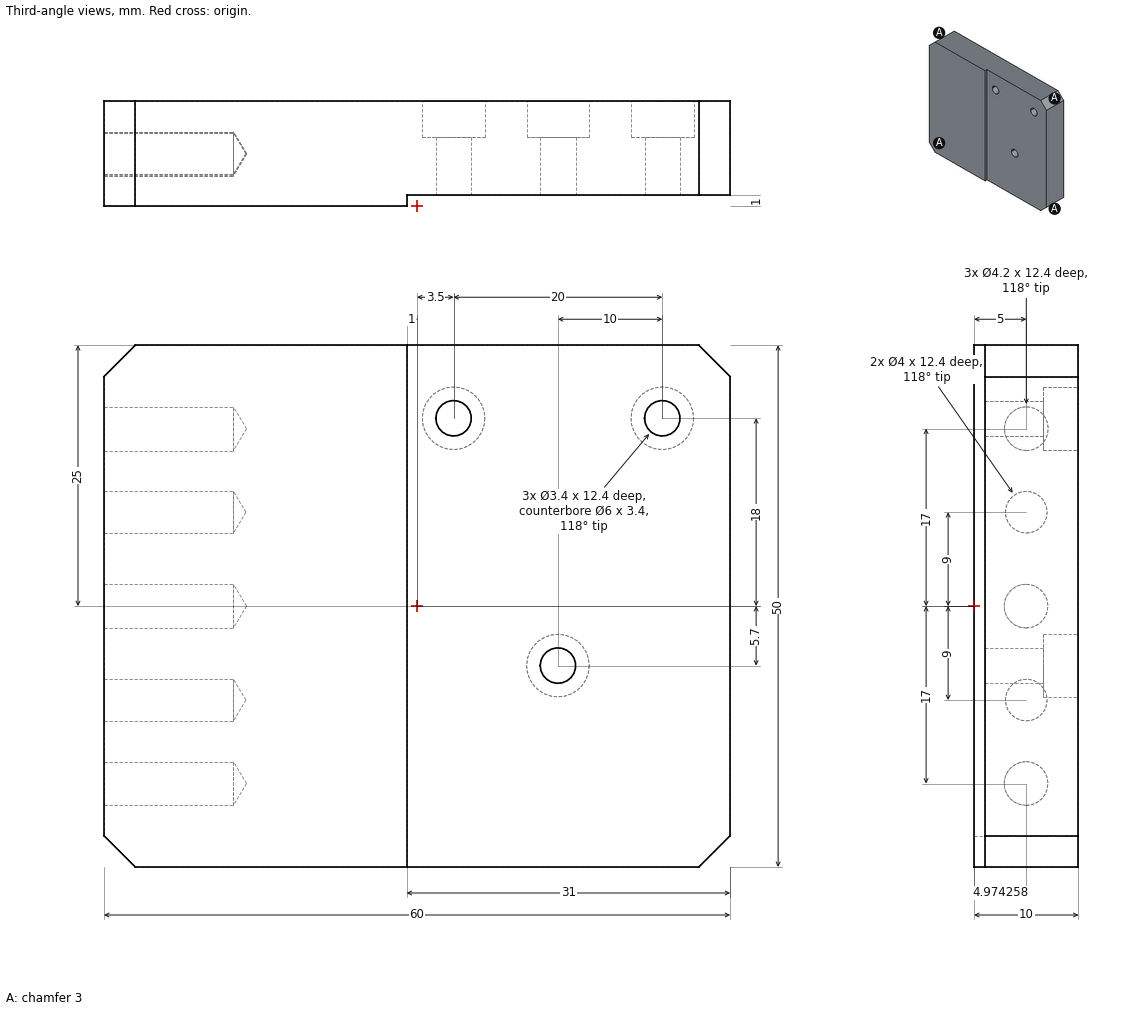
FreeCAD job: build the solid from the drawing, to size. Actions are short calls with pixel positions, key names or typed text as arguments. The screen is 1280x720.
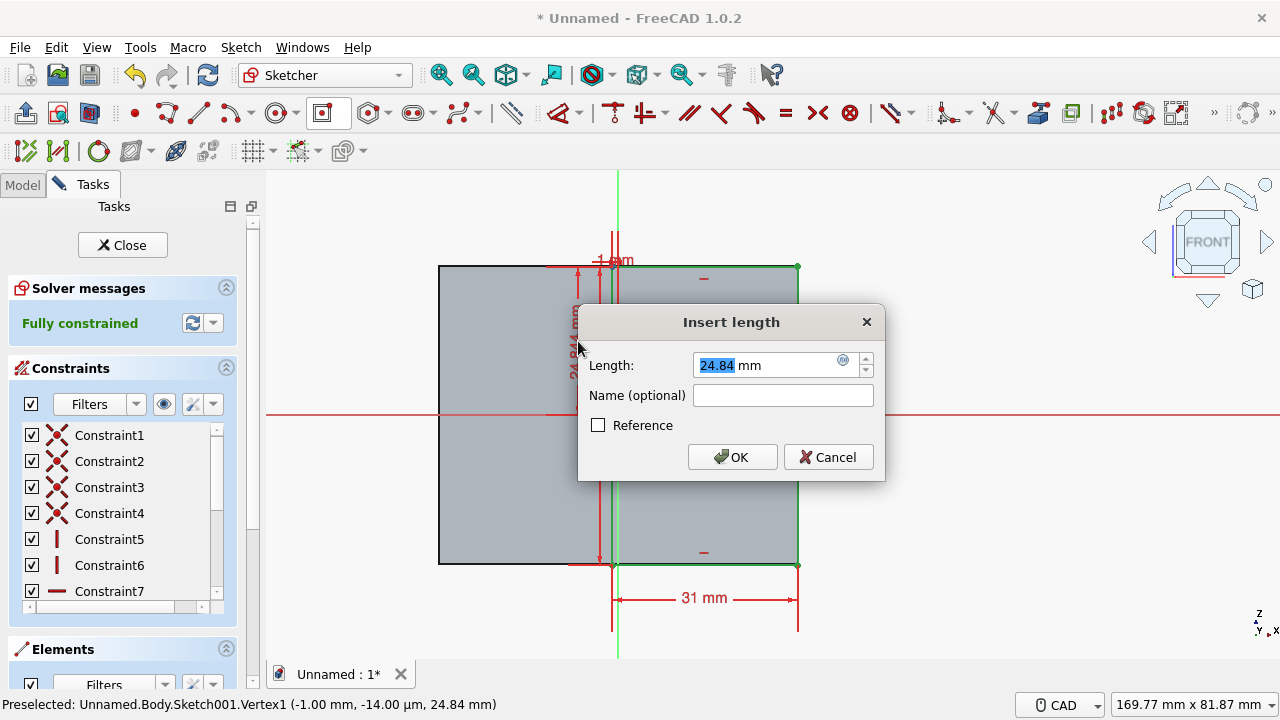
text(25)
key(Return)
key(Escape)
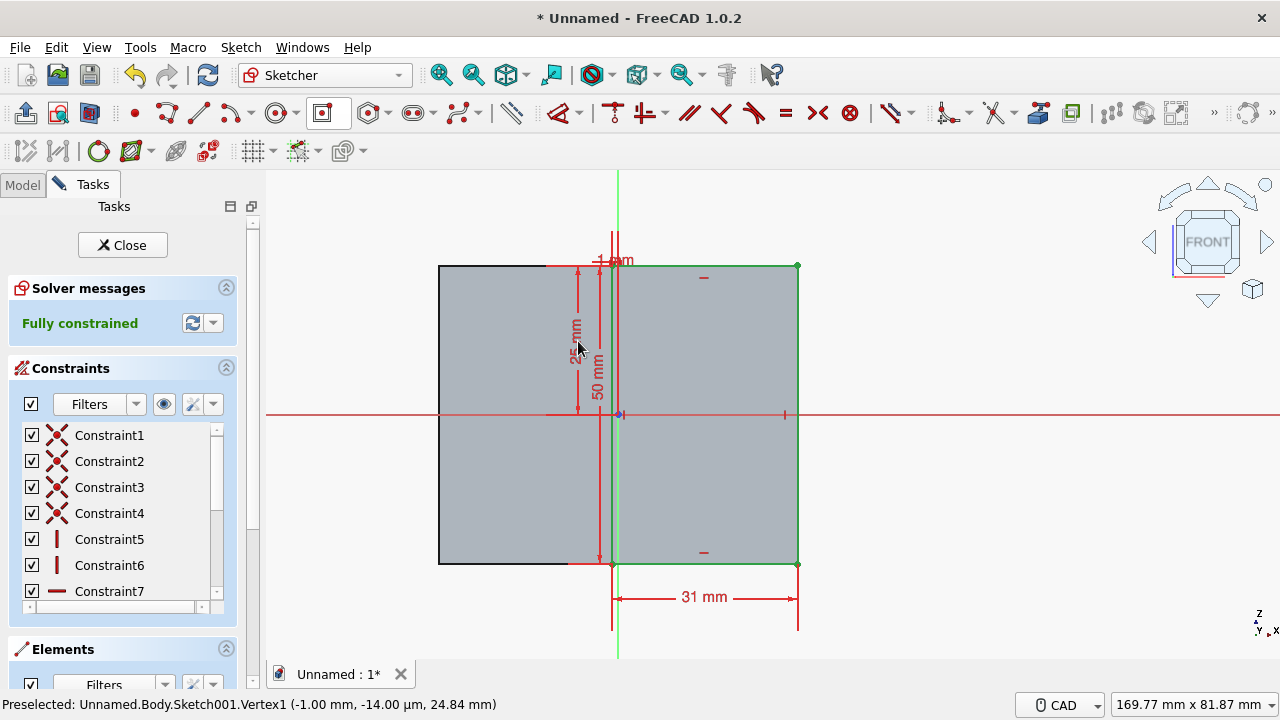
click(123, 245)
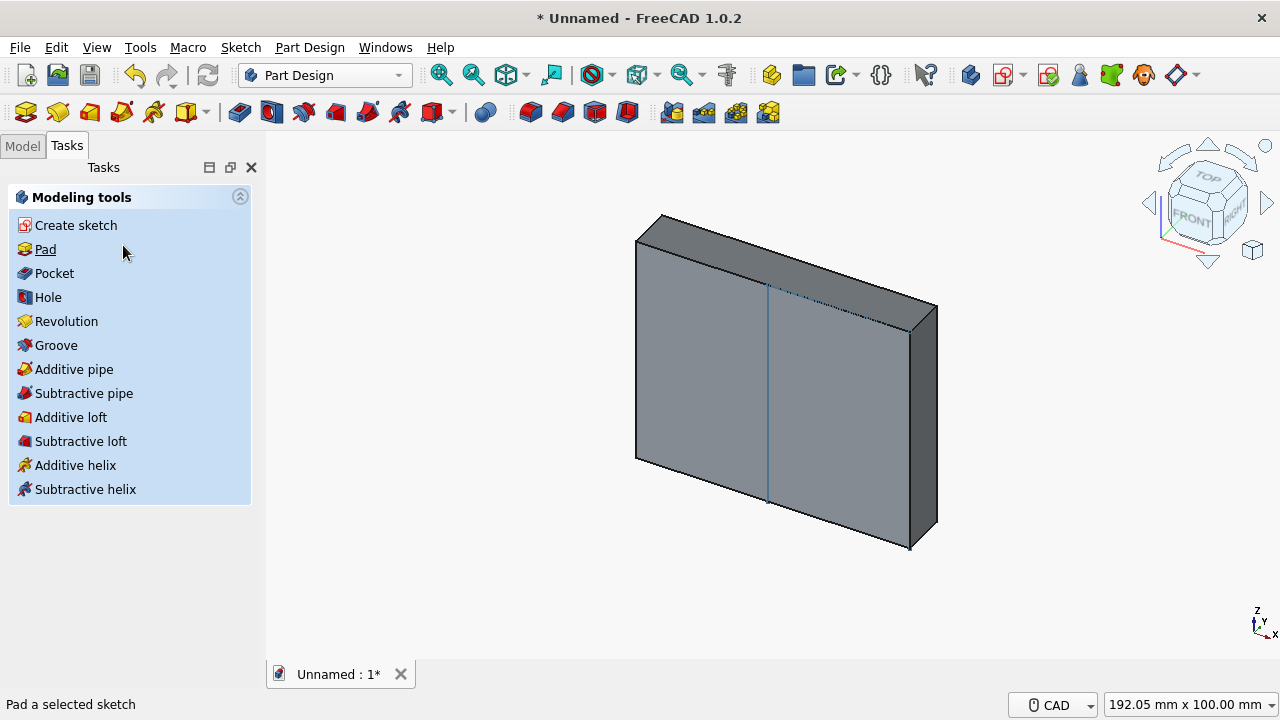
click(240, 112)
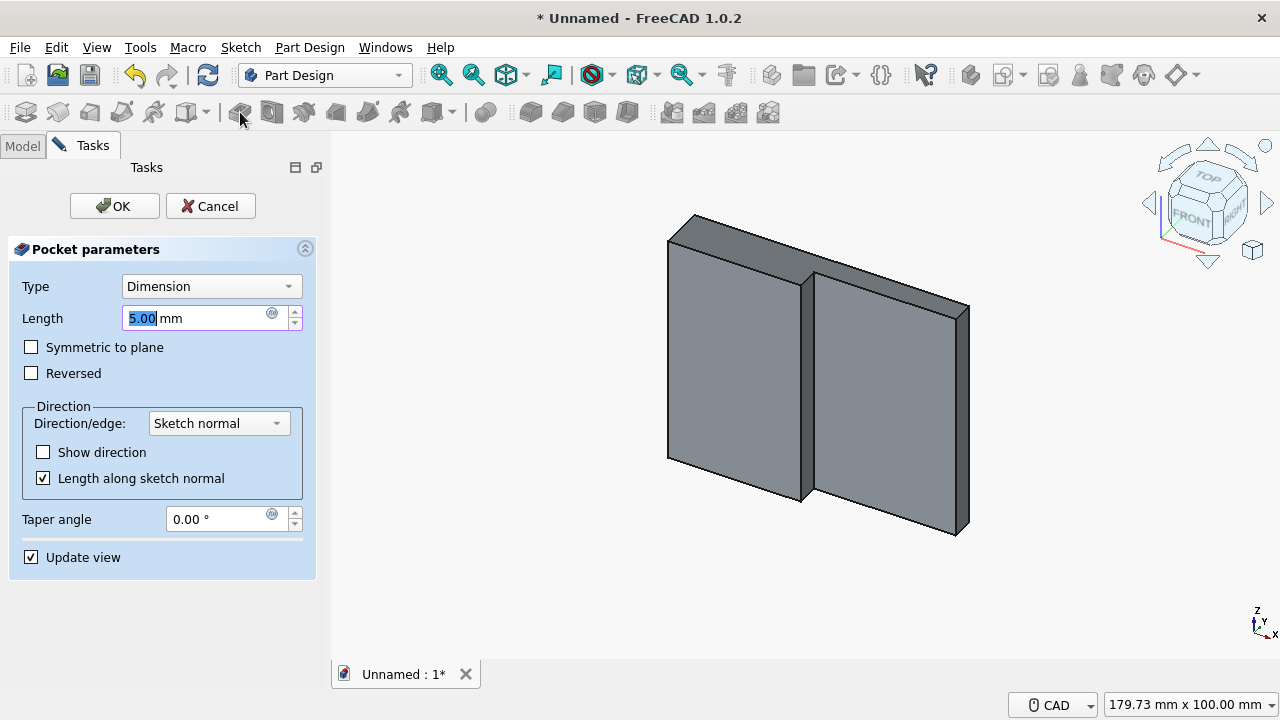
text(1)
key(Tab)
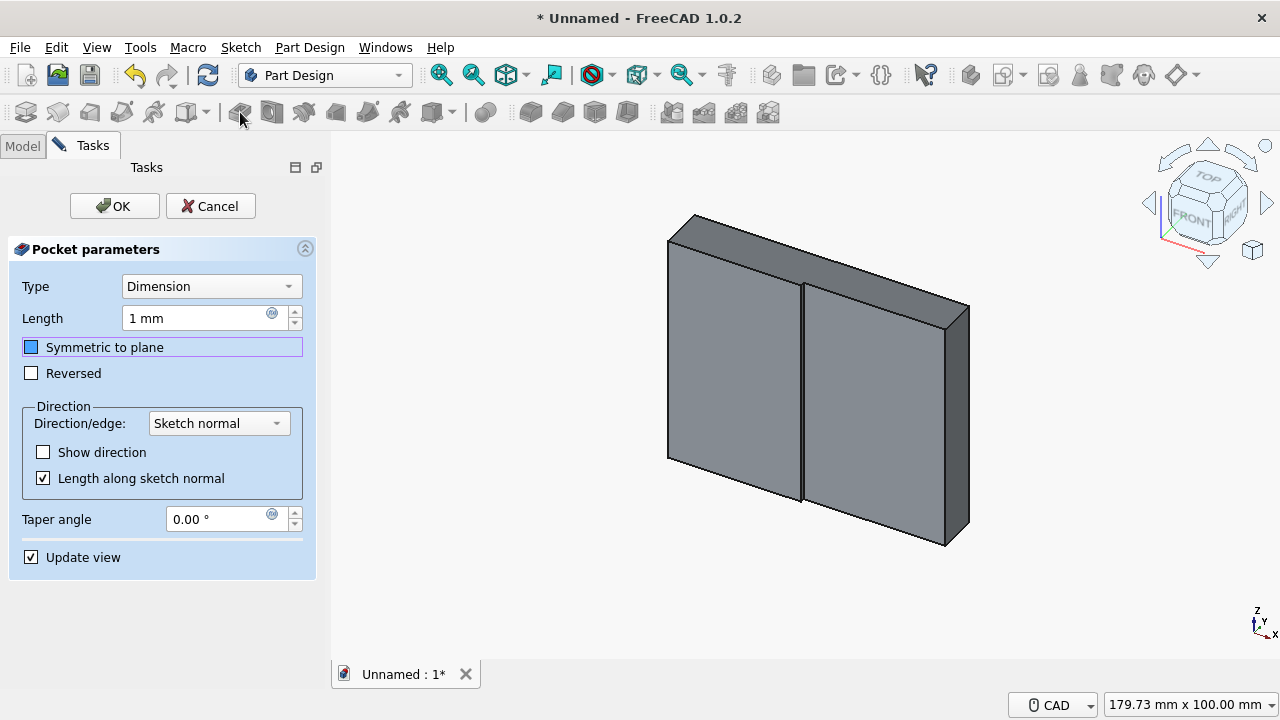
click(115, 206)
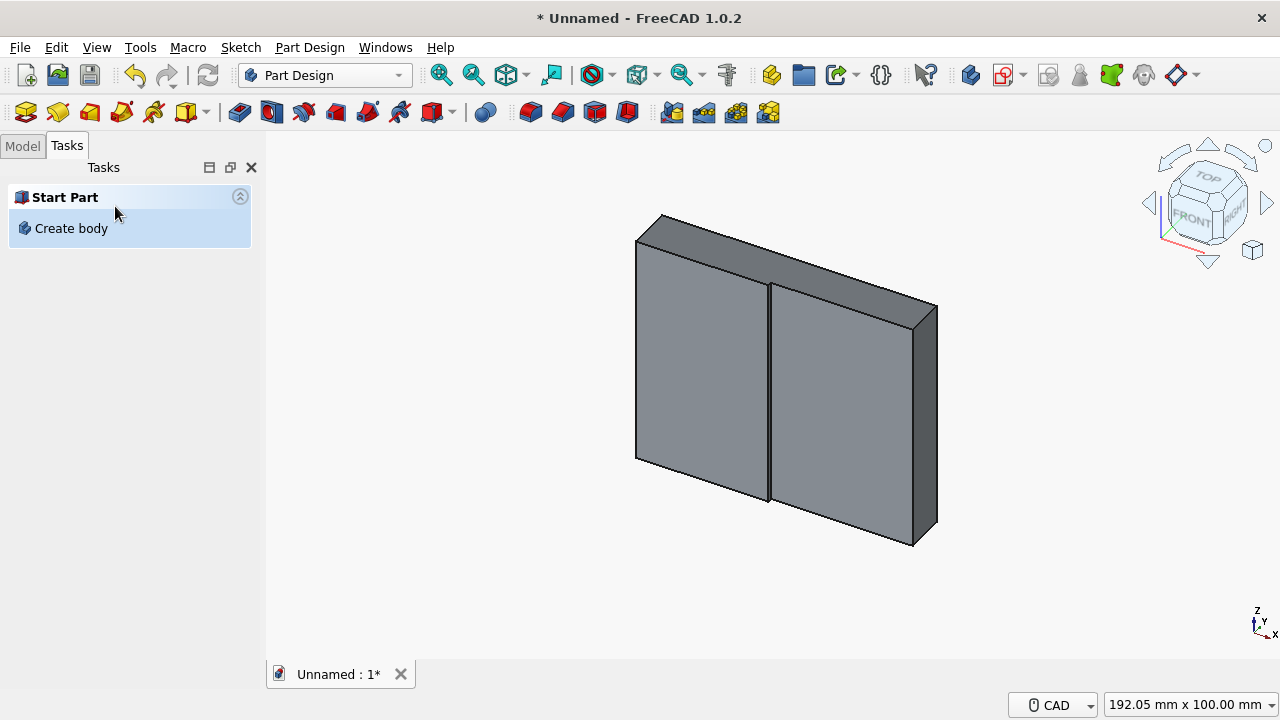
click(925, 317)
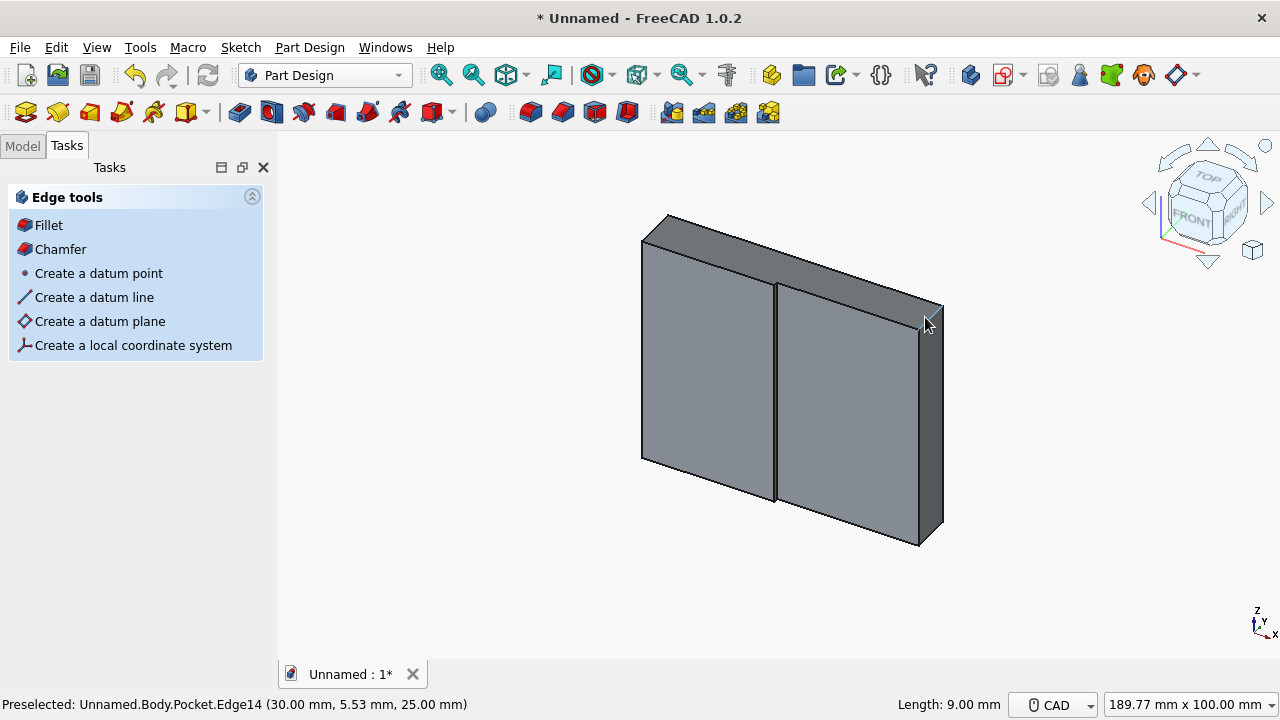
key(0)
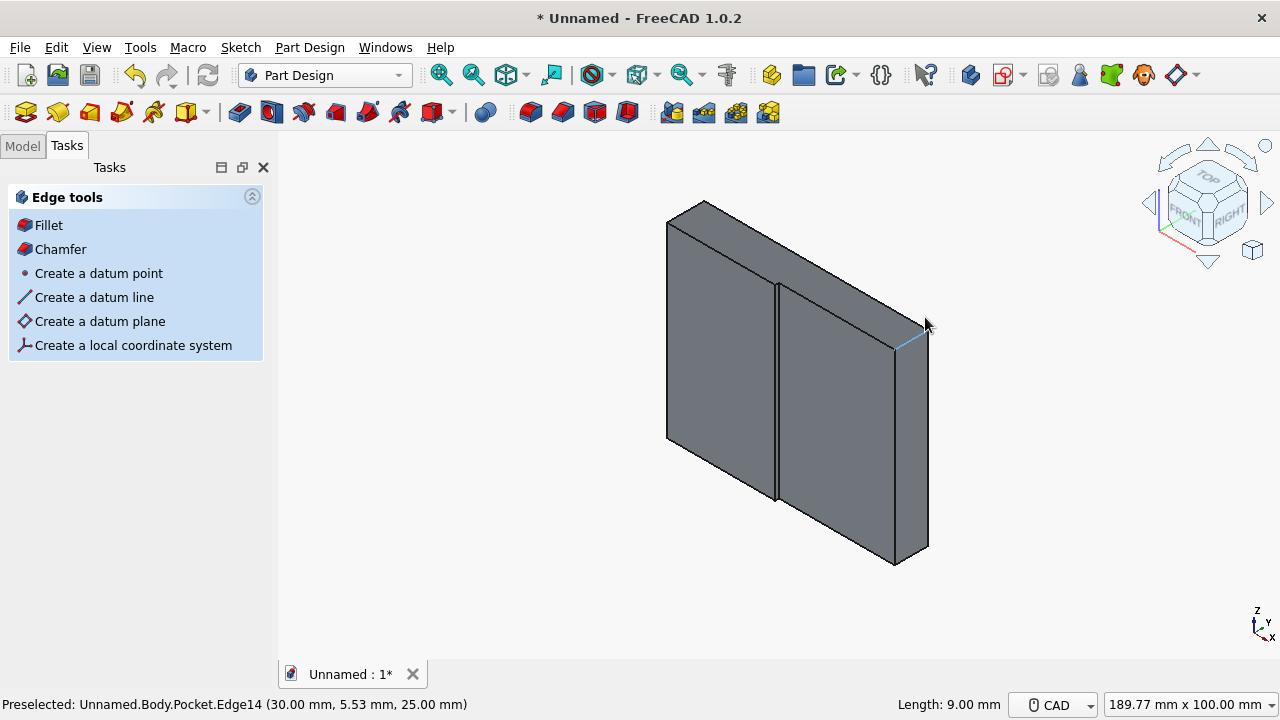
key(2)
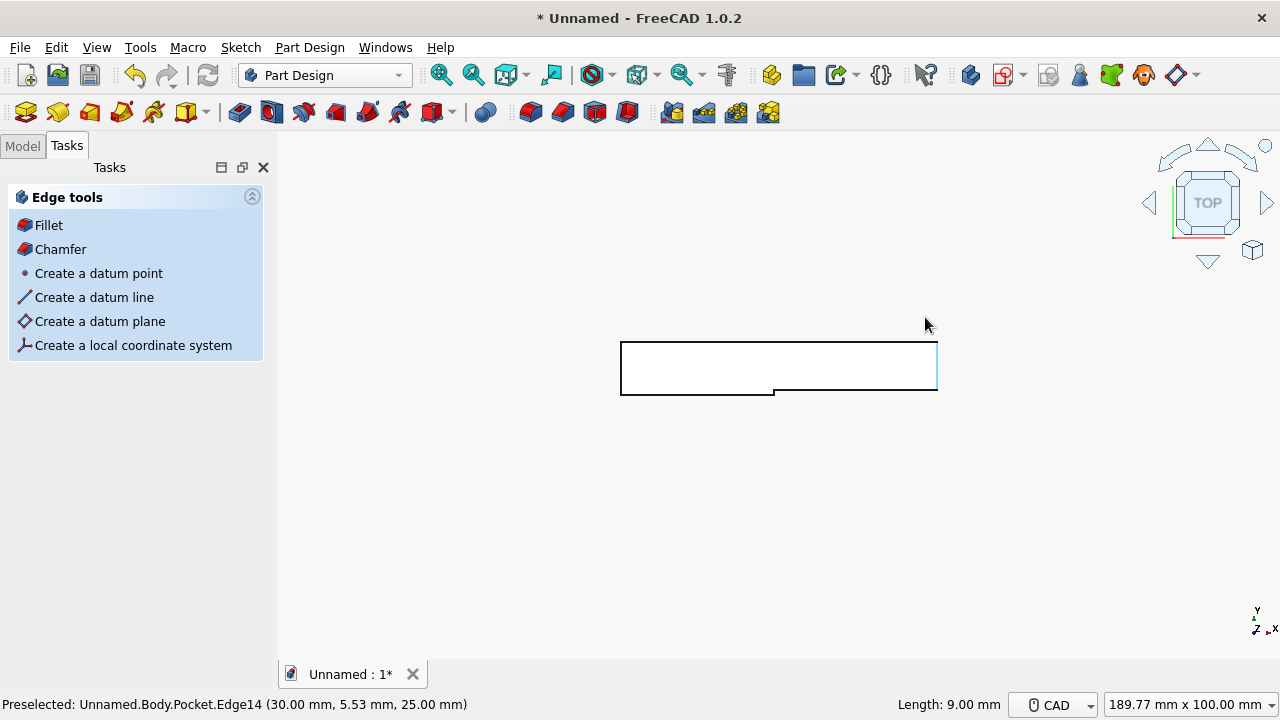
click(442, 76)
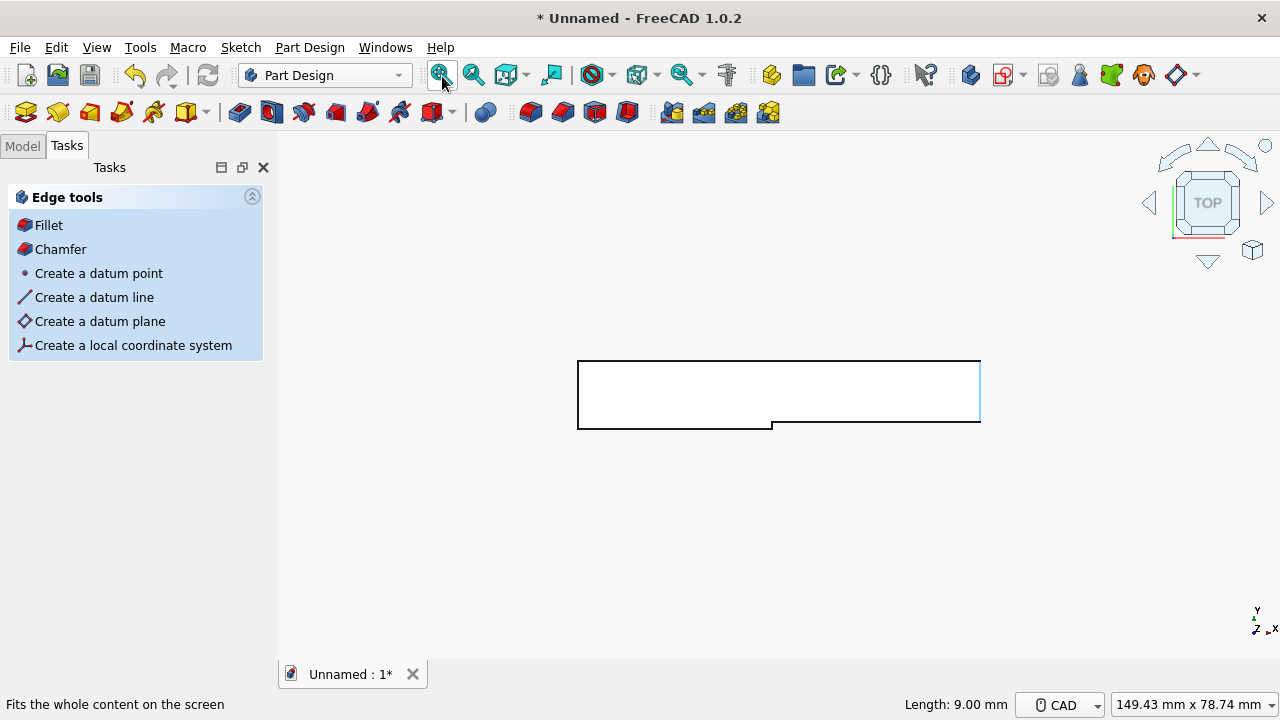
click(578, 394, ctrl)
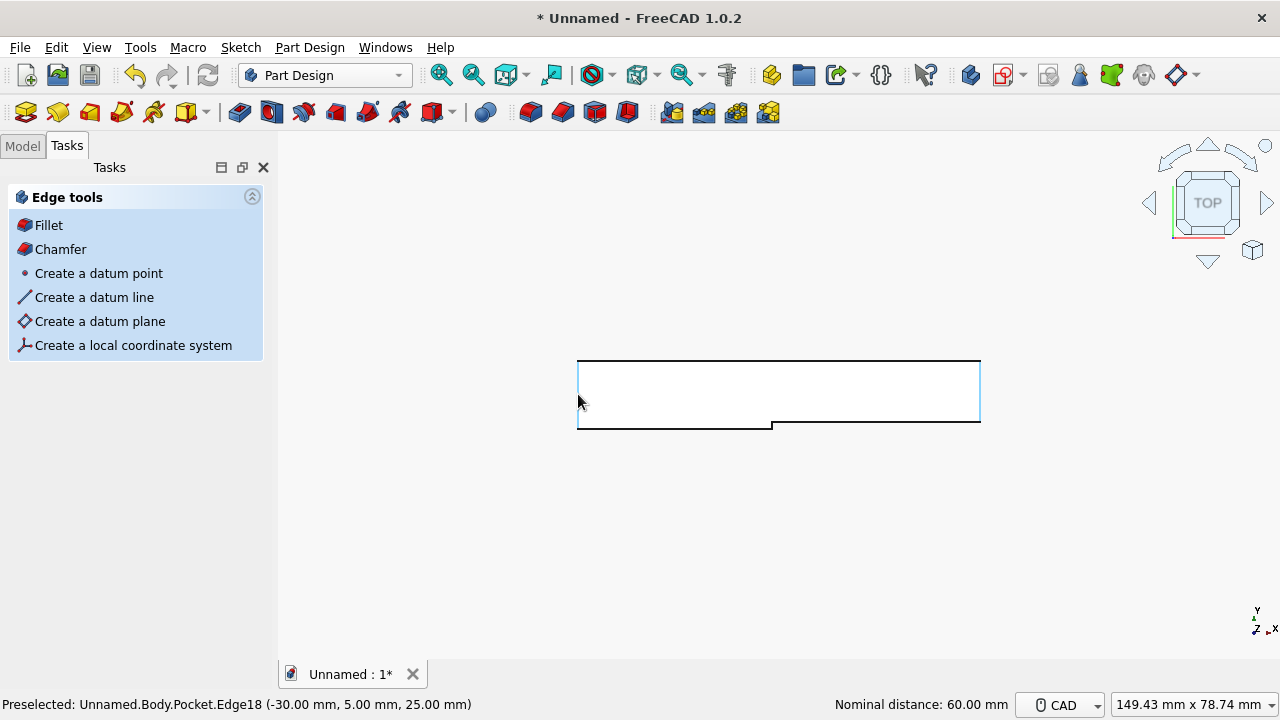
key(1)